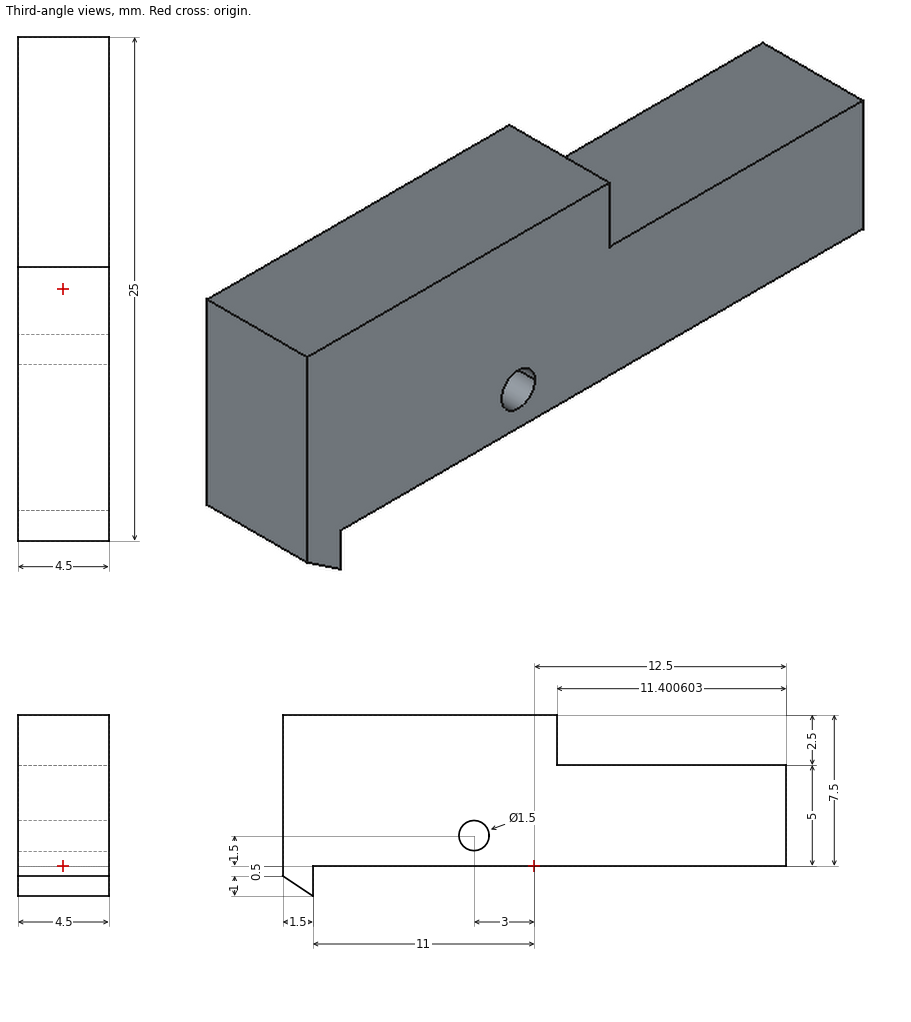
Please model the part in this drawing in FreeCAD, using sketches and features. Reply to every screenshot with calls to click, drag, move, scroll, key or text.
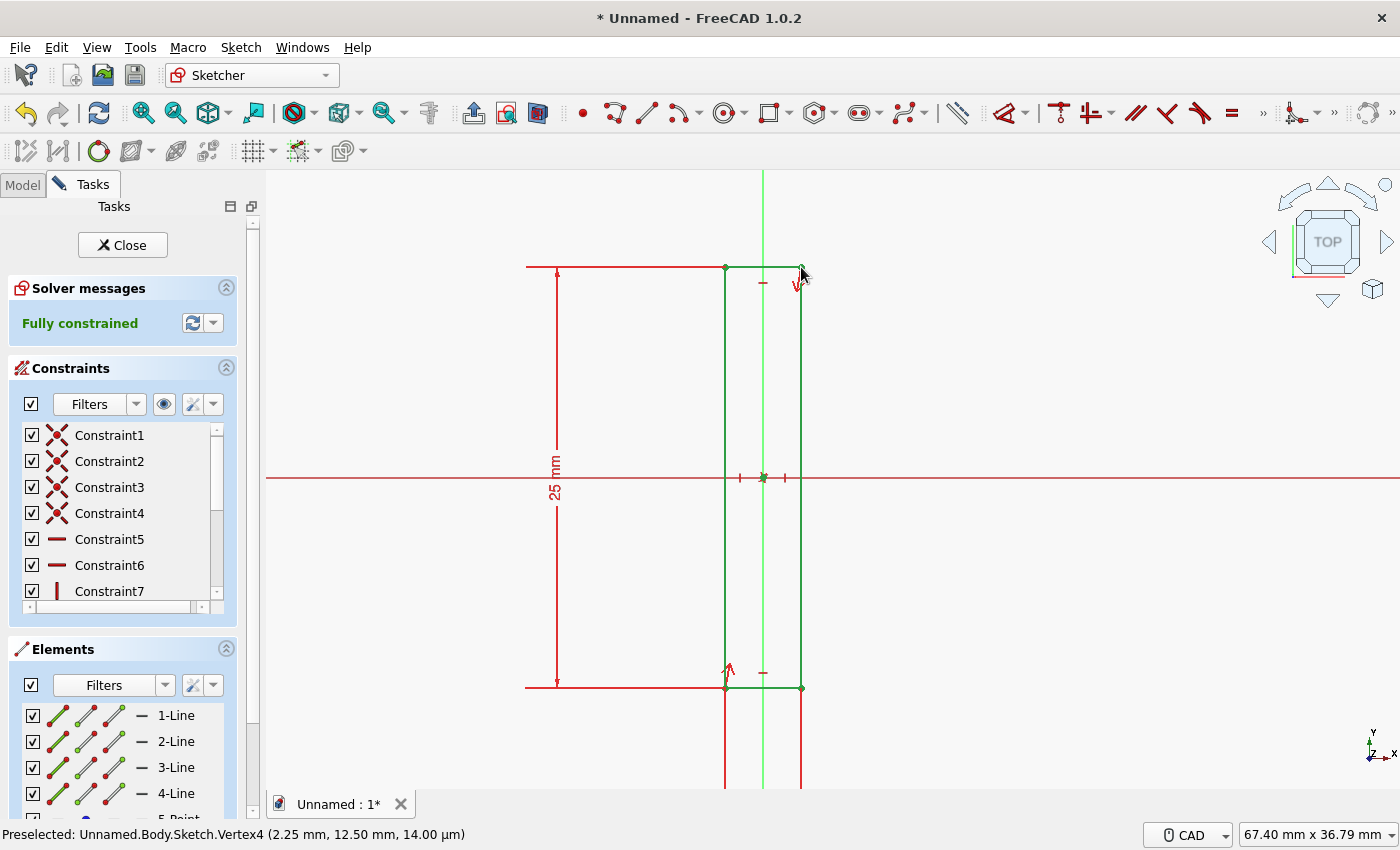
click(123, 245)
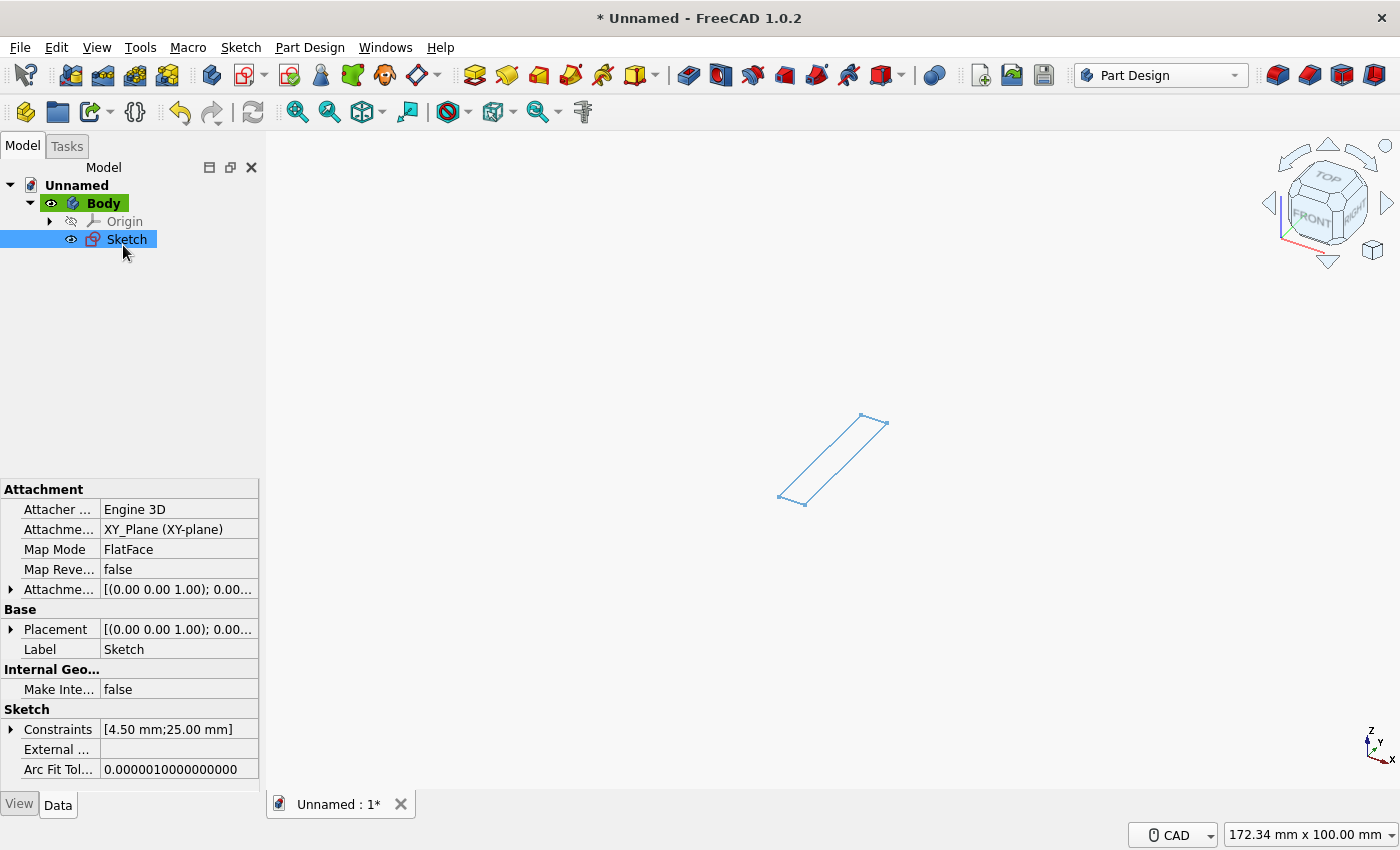
click(476, 76)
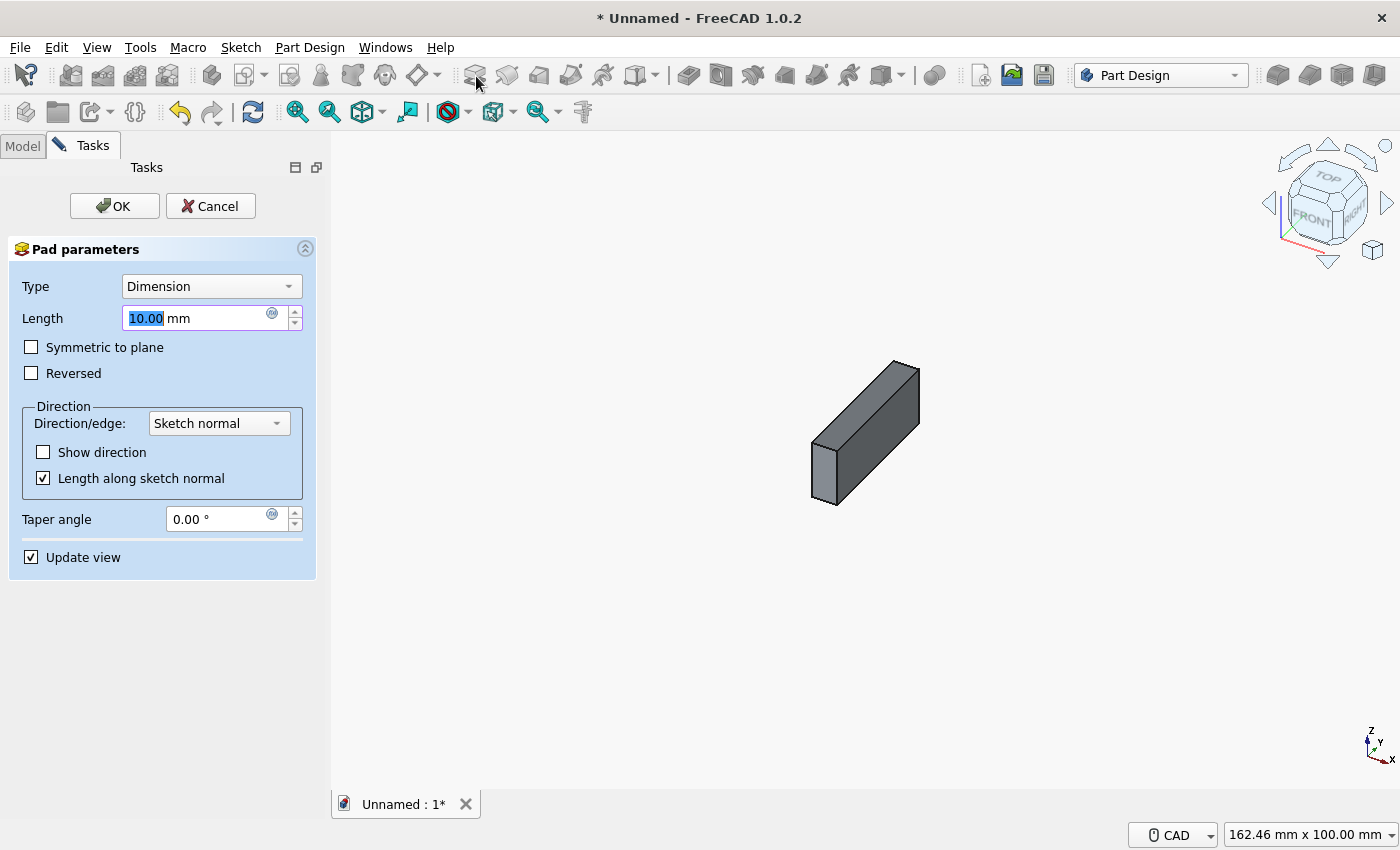
text(7.5)
key(Tab)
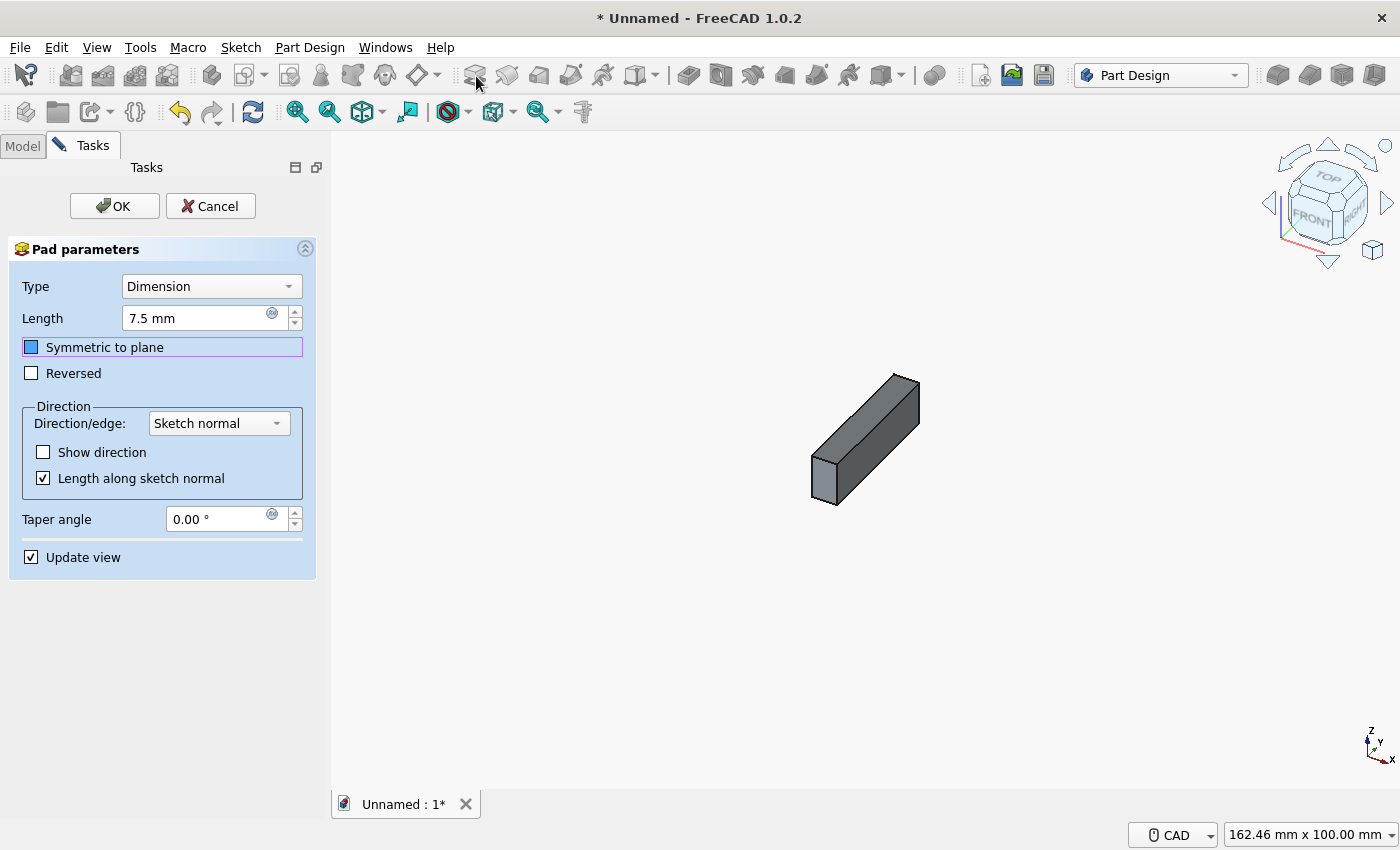
click(115, 206)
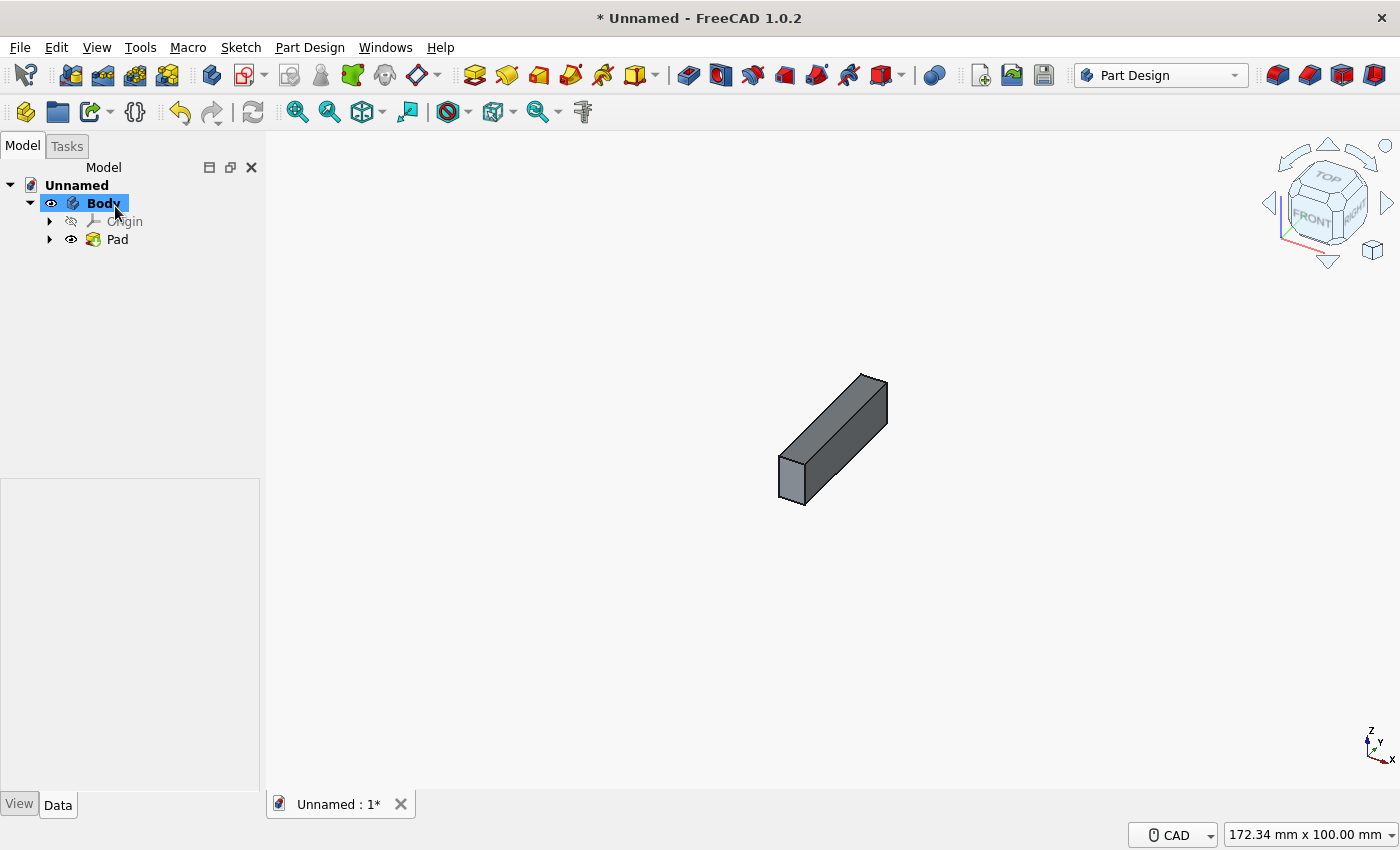
key(v)
key(f)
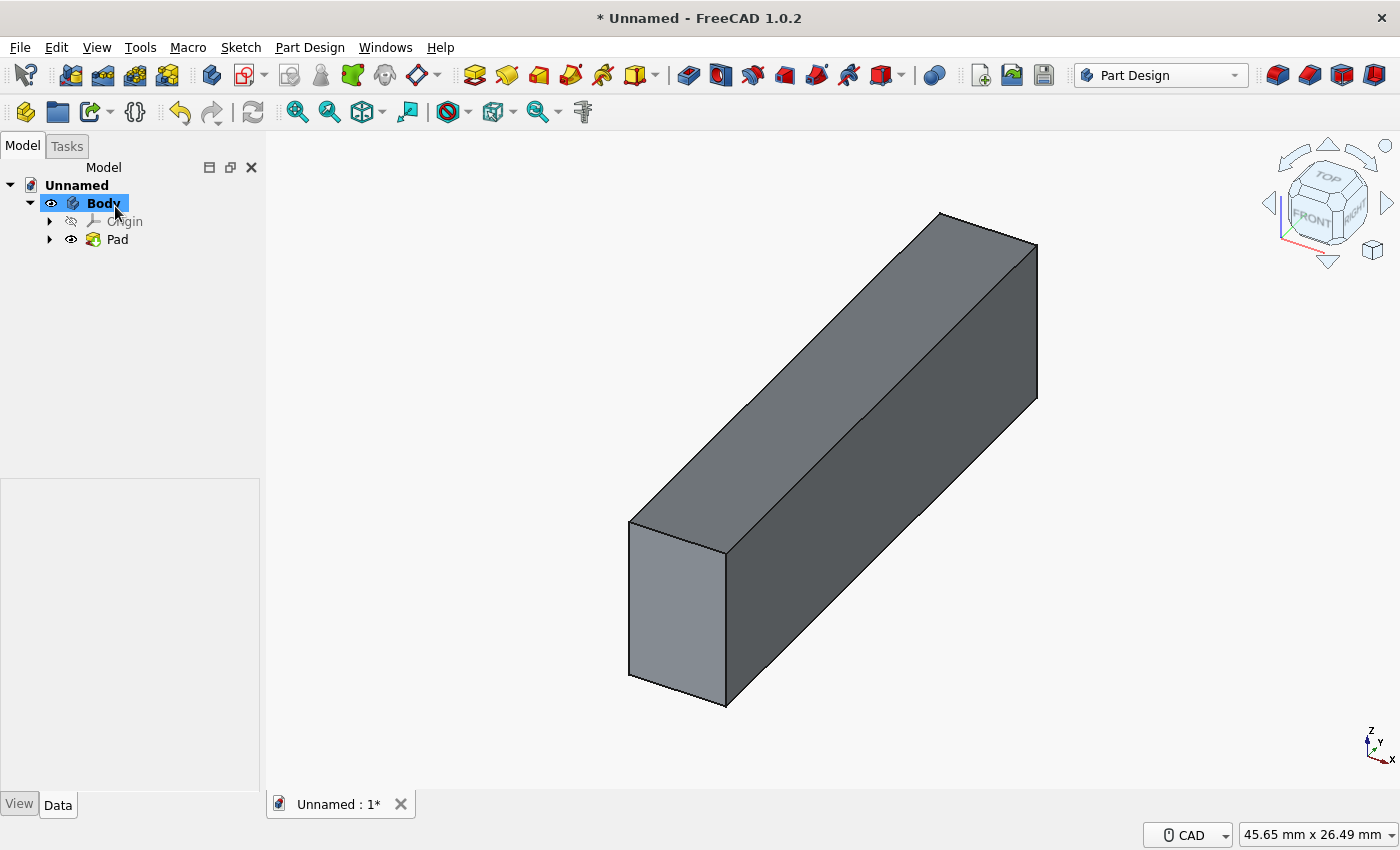
click(970, 387)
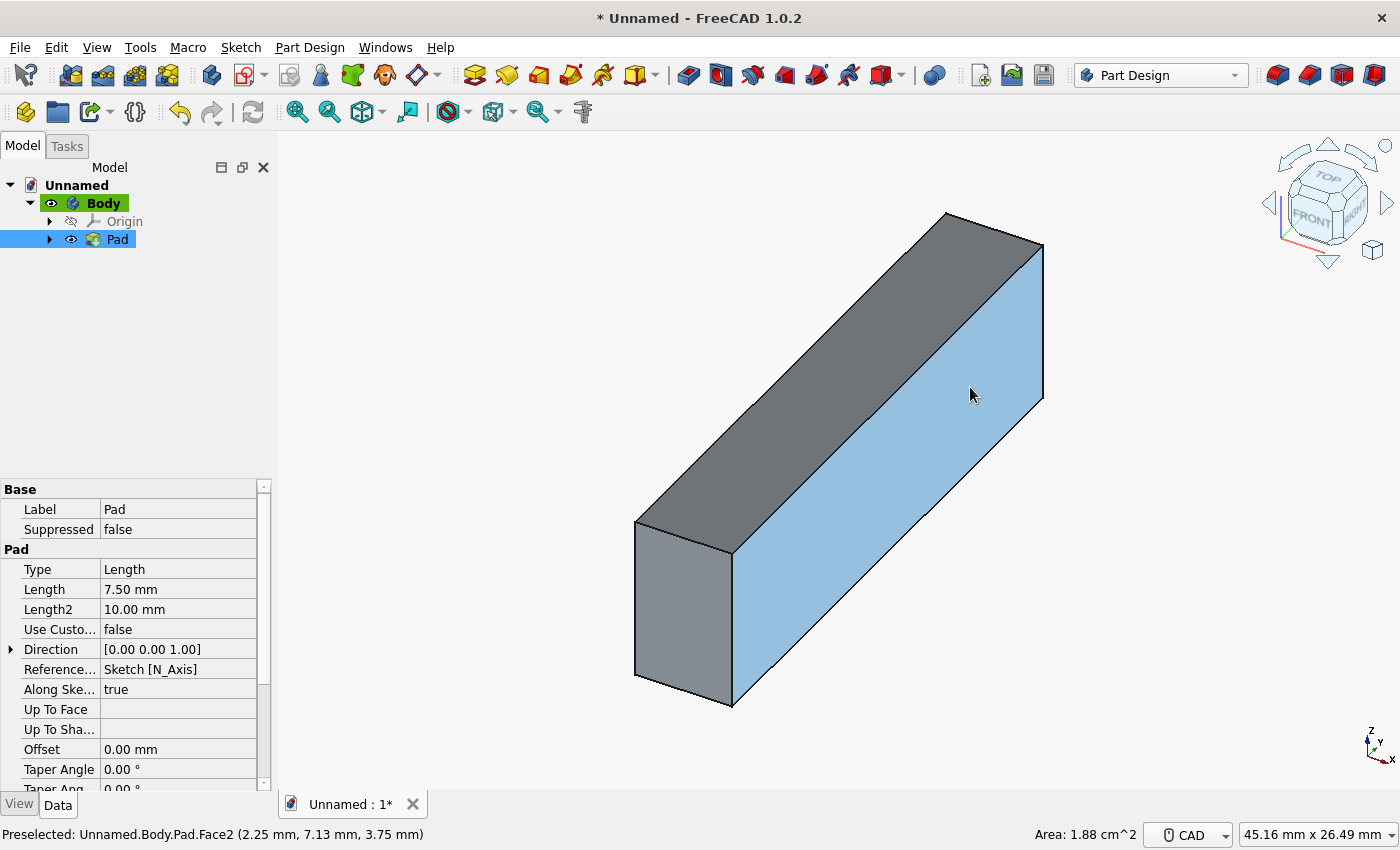
click(244, 76)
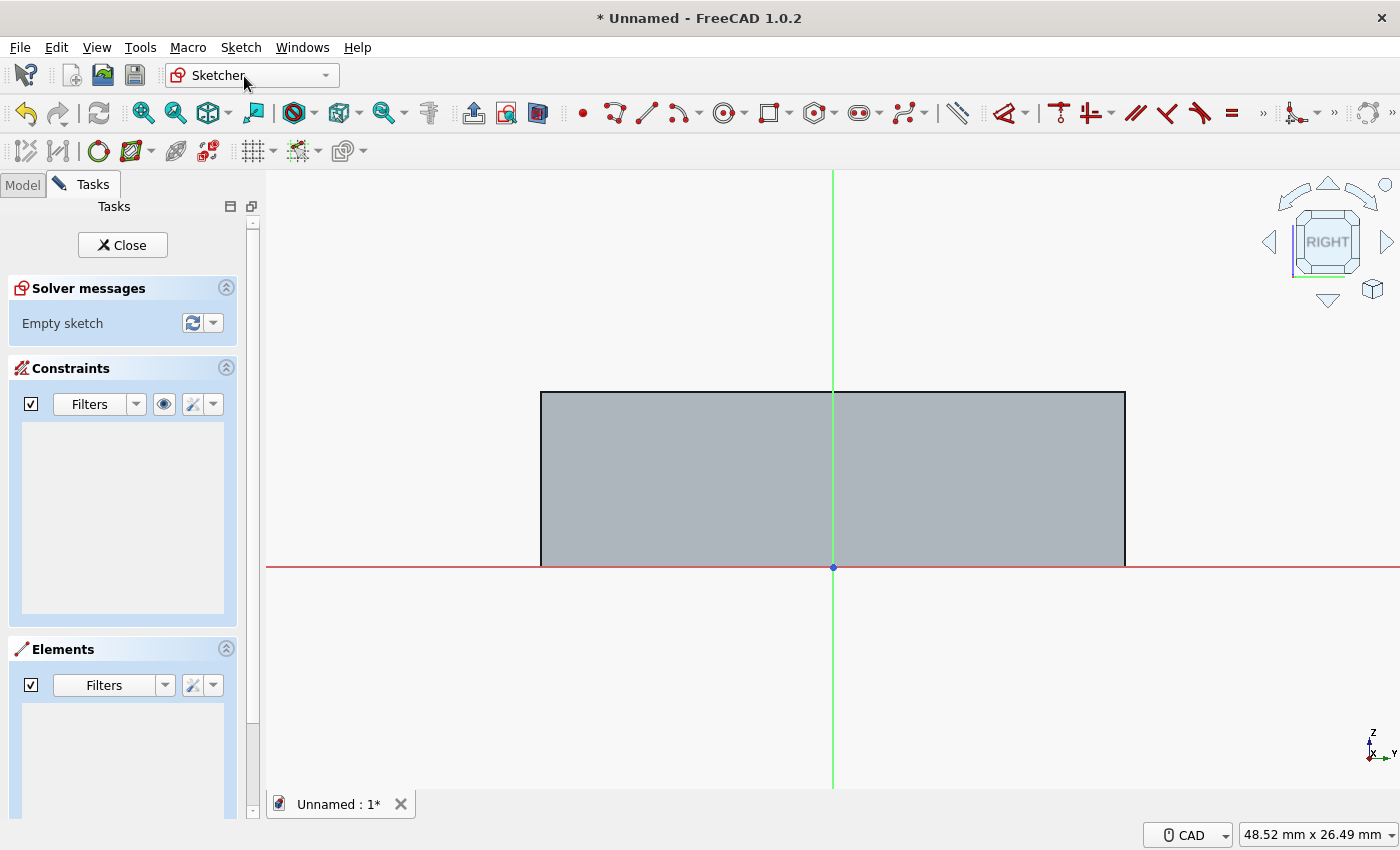
scroll(538, 595, up, 12)